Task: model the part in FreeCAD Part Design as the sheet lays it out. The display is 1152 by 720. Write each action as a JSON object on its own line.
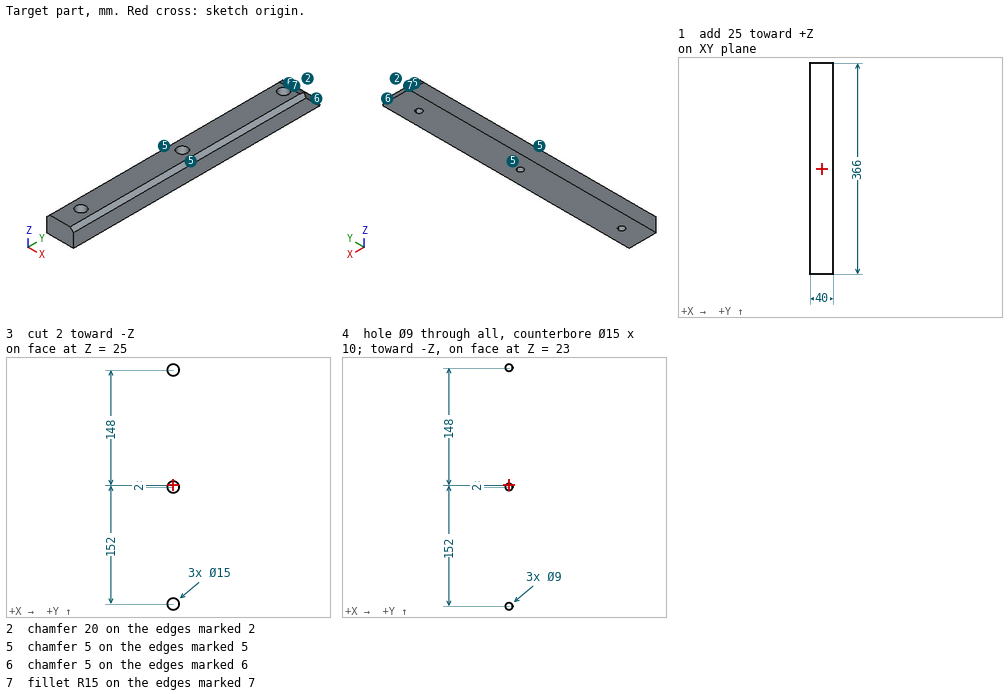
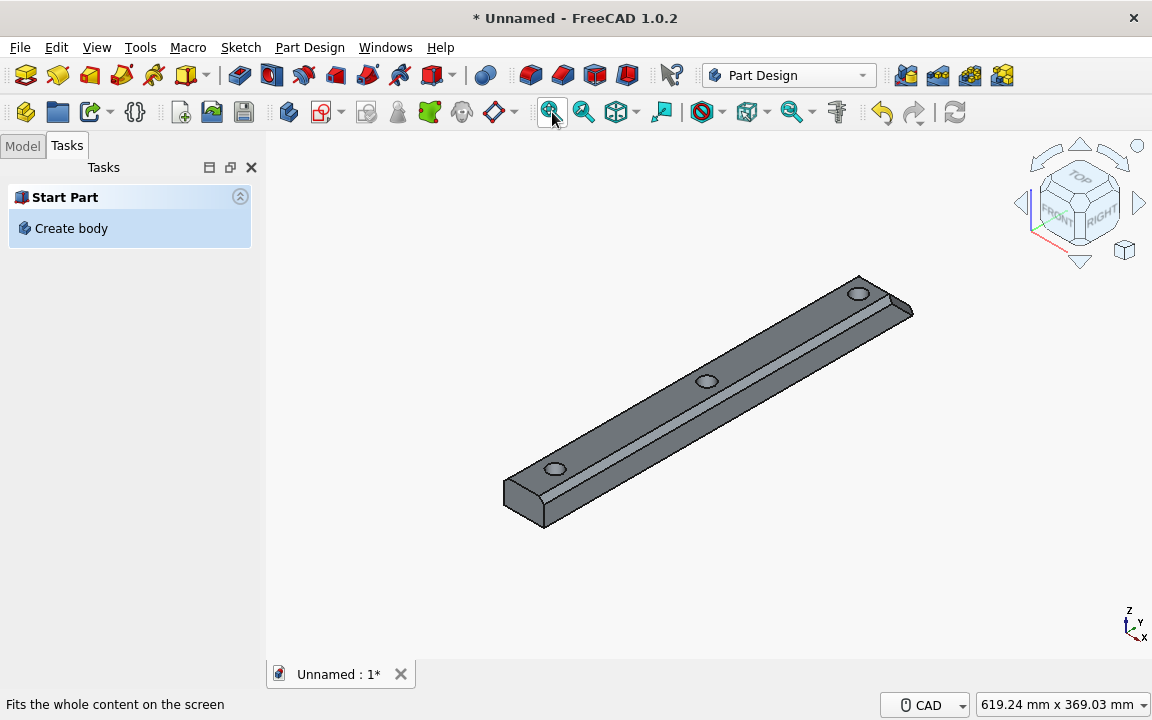
{"action": "key", "text": "2"}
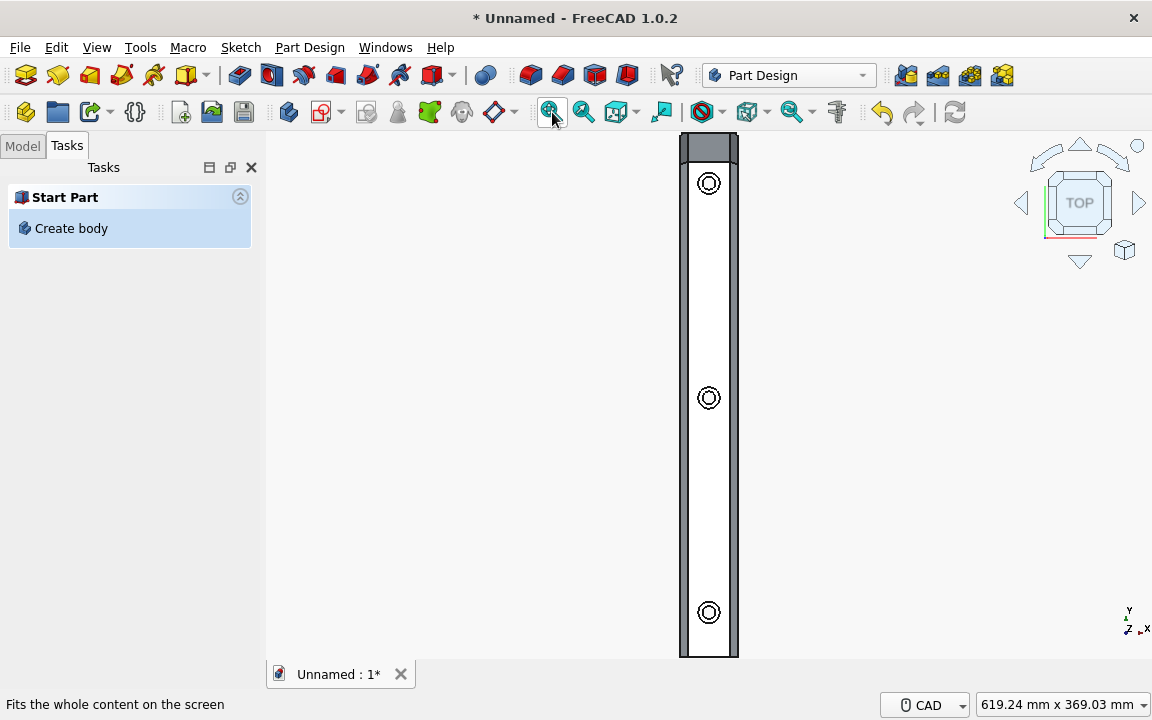
{"action": "left_click", "coordinate": [709, 161]}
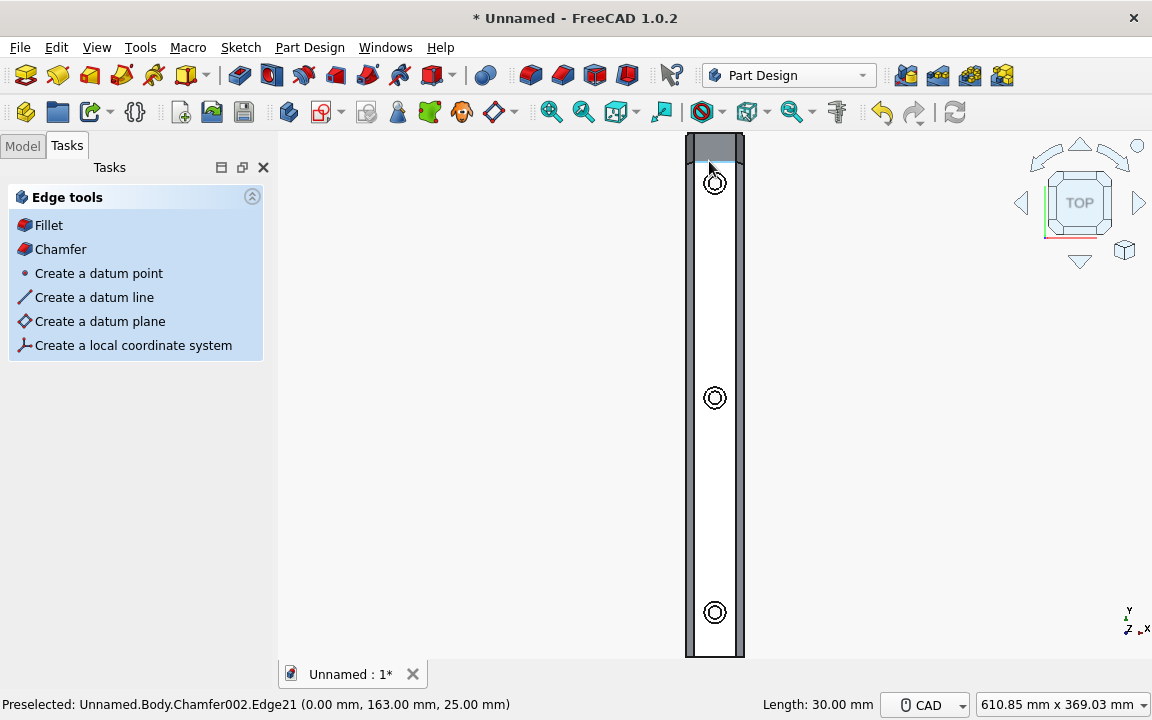
{"action": "left_click", "coordinate": [532, 76]}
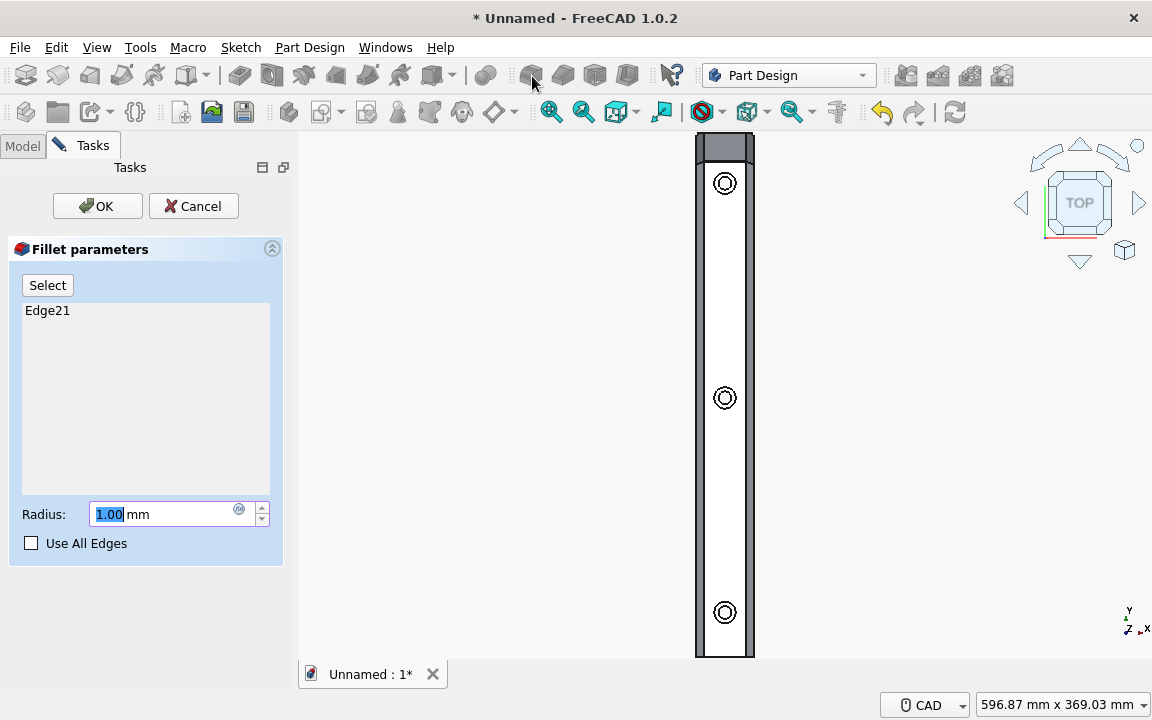
{"action": "type", "text": "15"}
{"action": "key", "text": "Tab"}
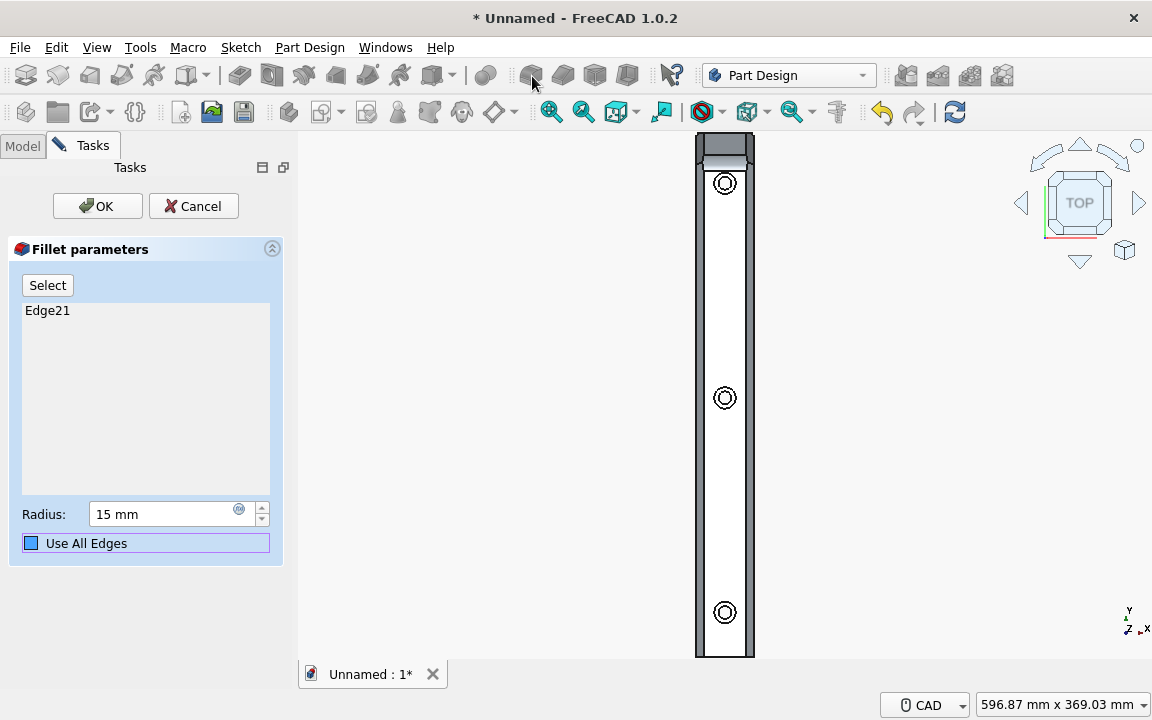
{"action": "left_click", "coordinate": [98, 206]}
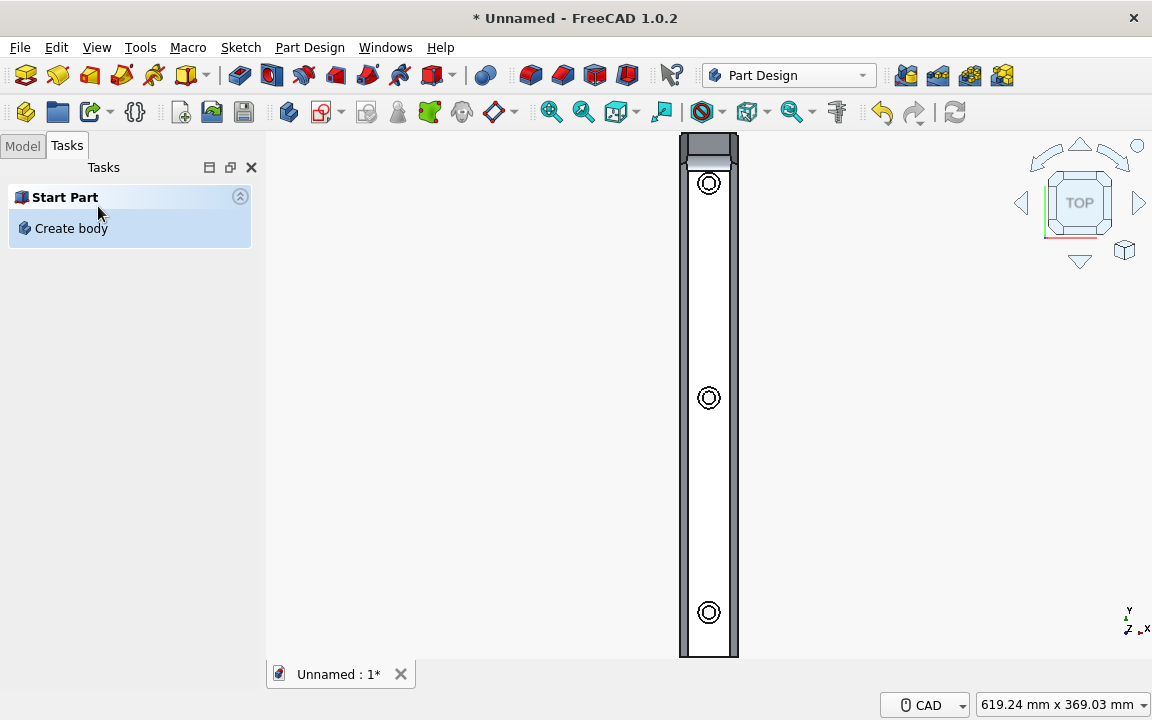
{"action": "key", "text": "0"}